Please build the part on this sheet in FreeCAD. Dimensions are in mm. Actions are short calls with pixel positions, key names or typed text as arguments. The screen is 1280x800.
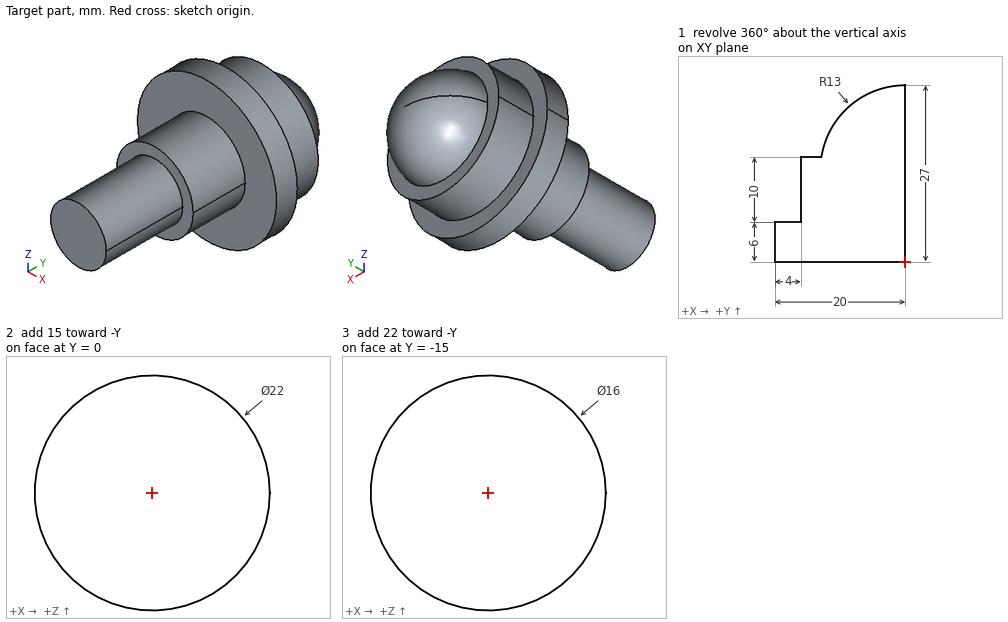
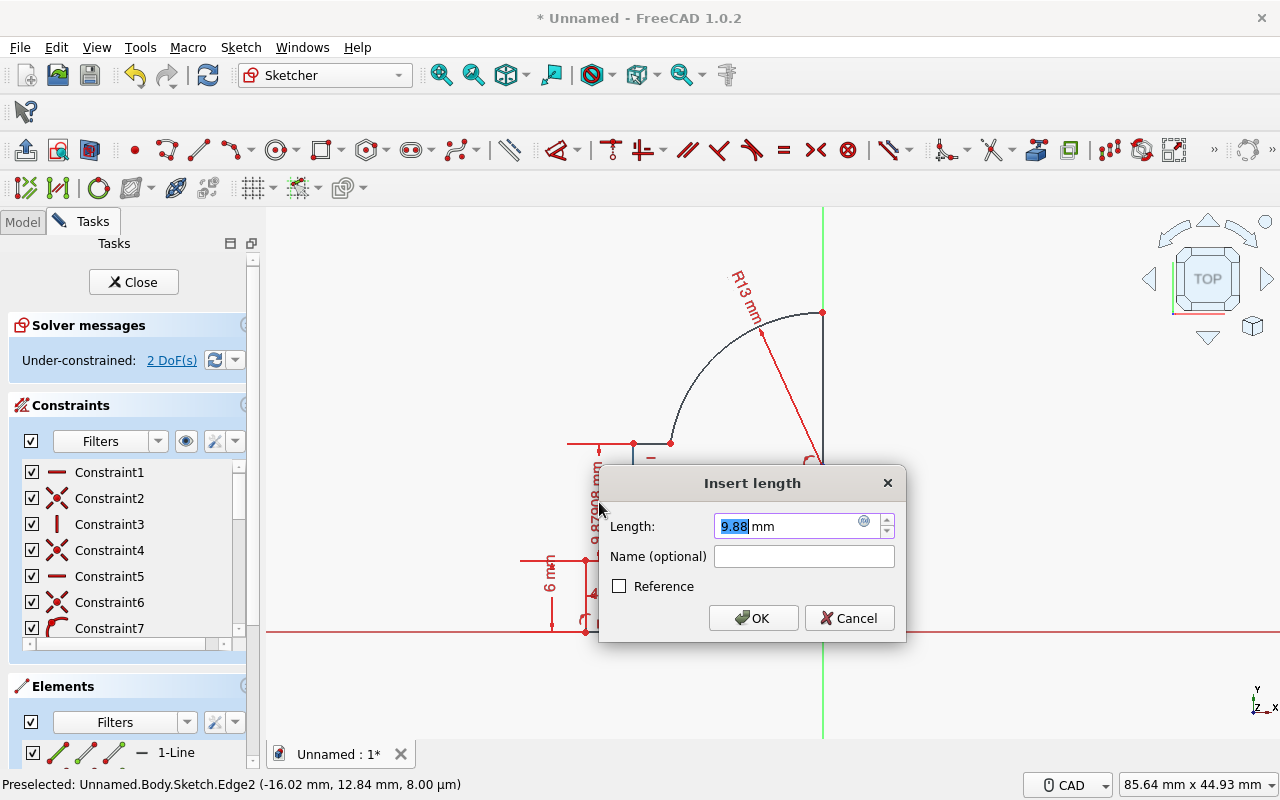
text(10)
key(Return)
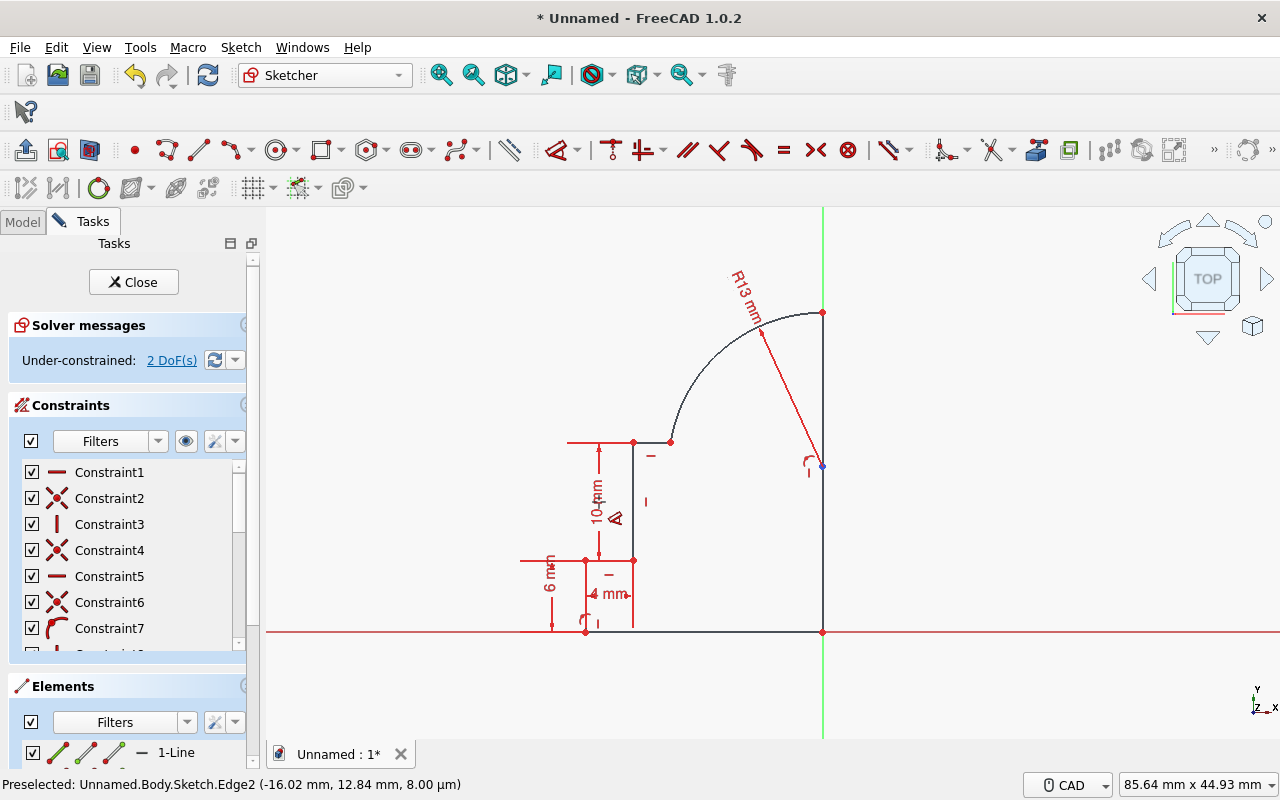
click(657, 632)
click(704, 666)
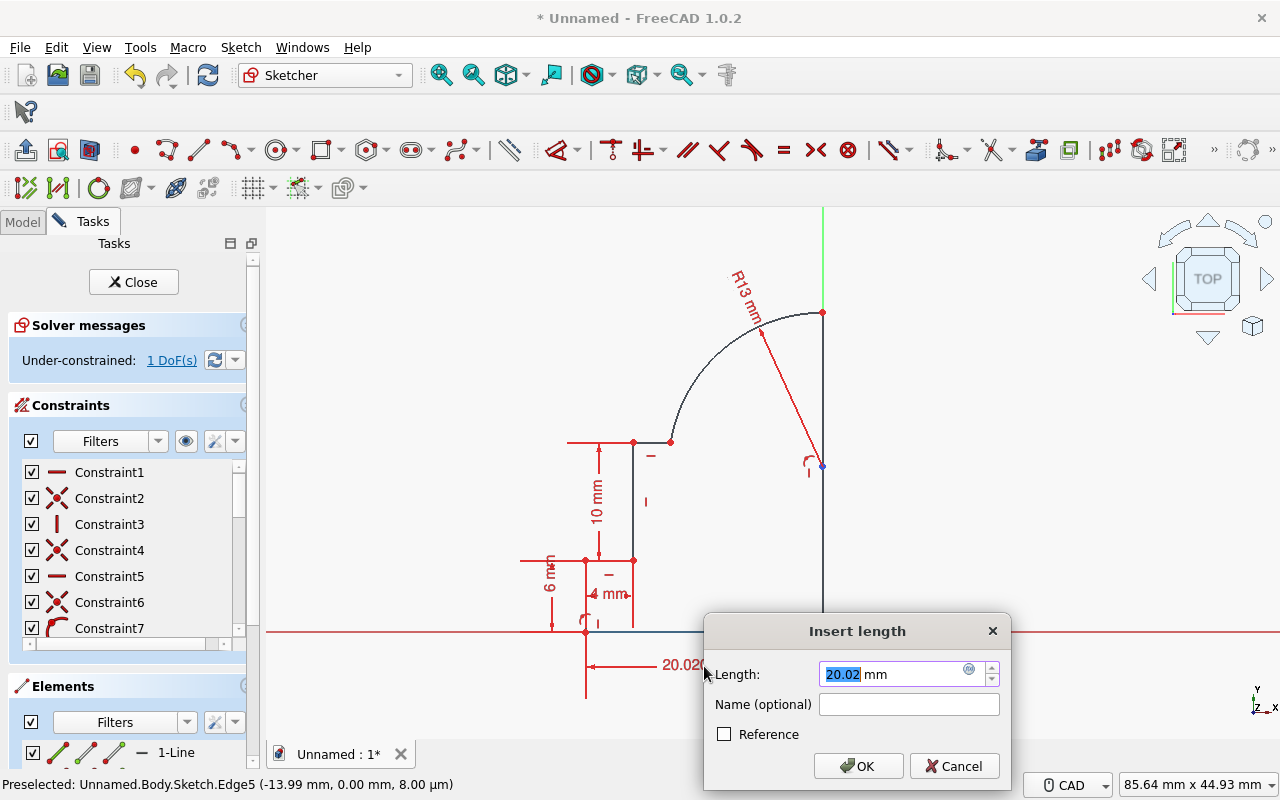
text(20)
key(Return)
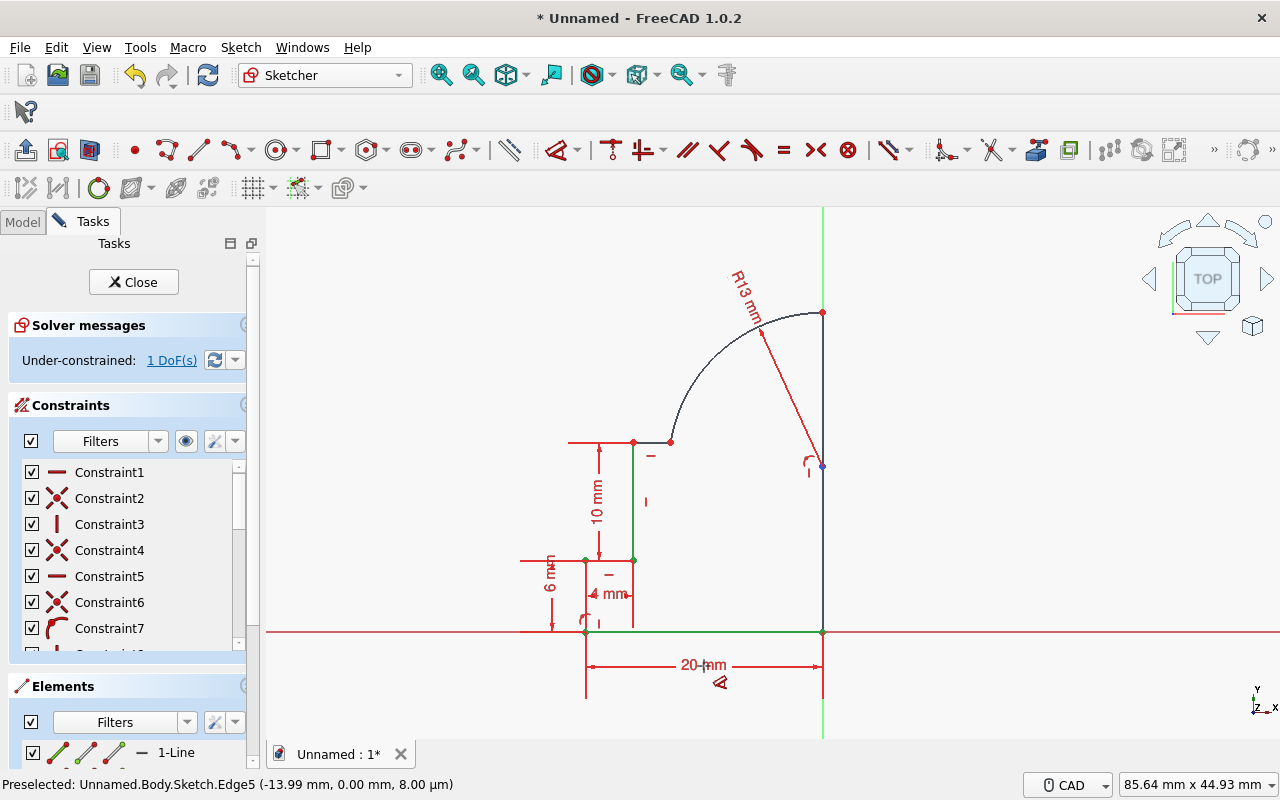
click(823, 536)
click(857, 472)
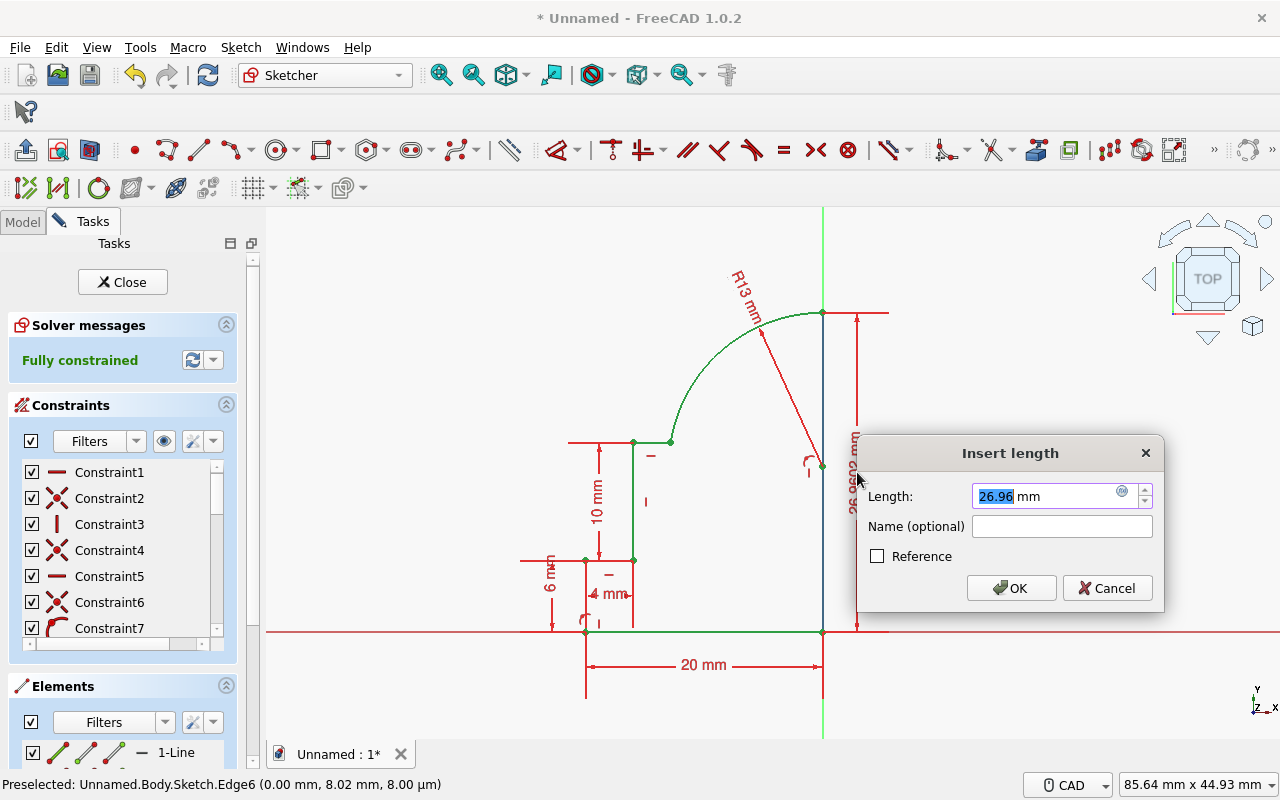
text(27)
key(Return)
key(Escape)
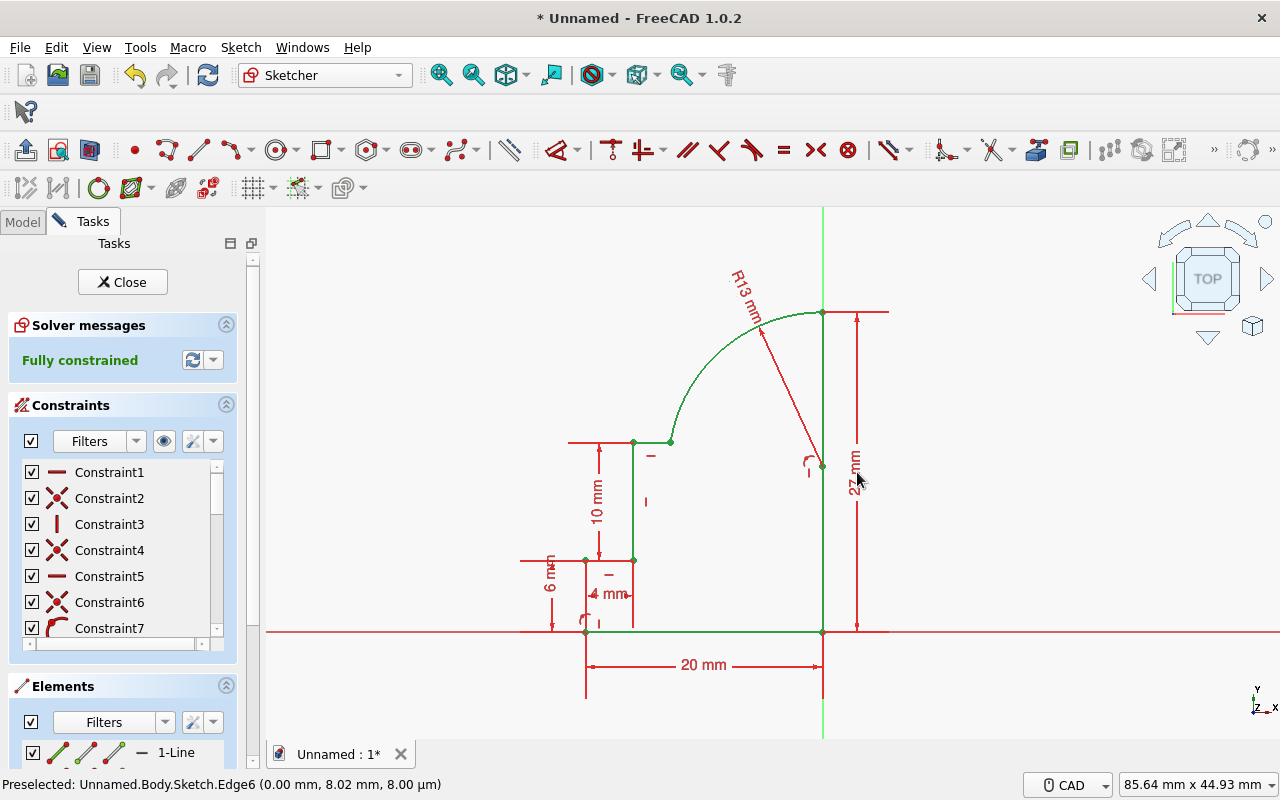
click(123, 282)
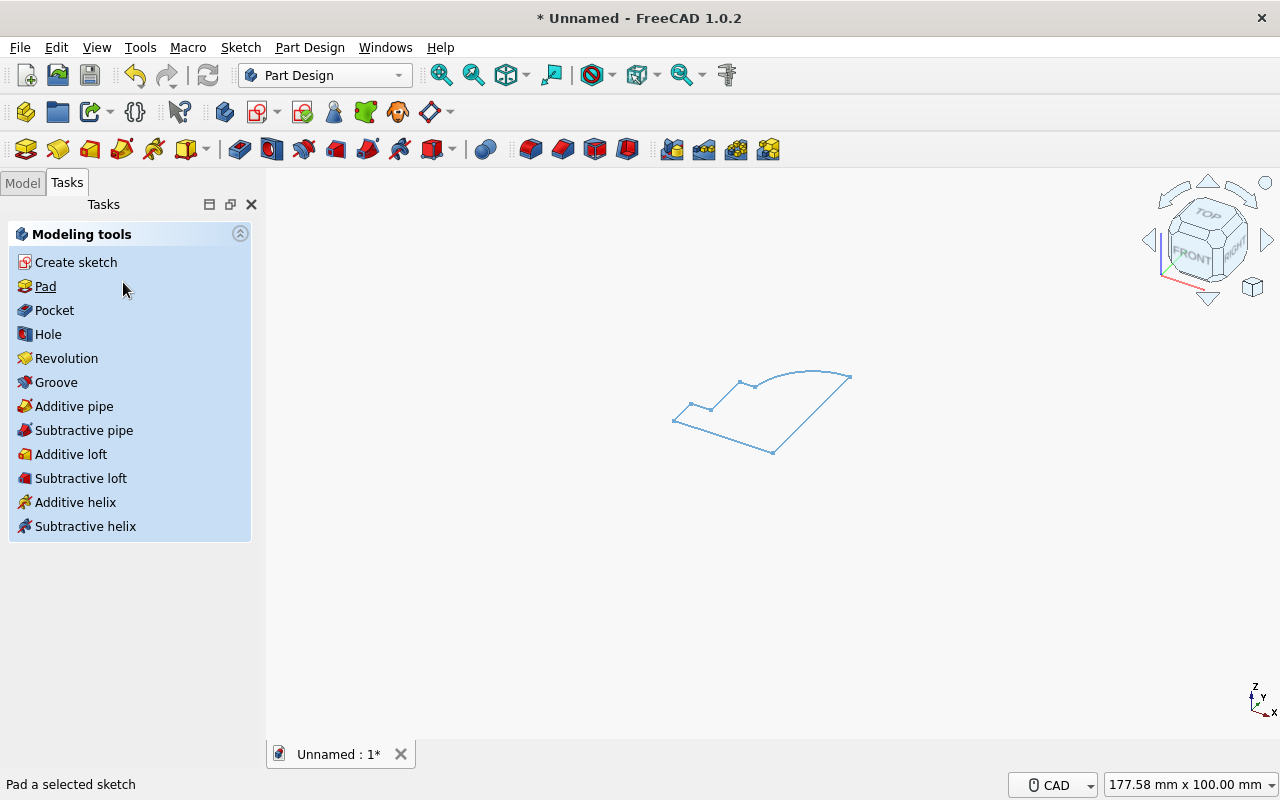
click(58, 150)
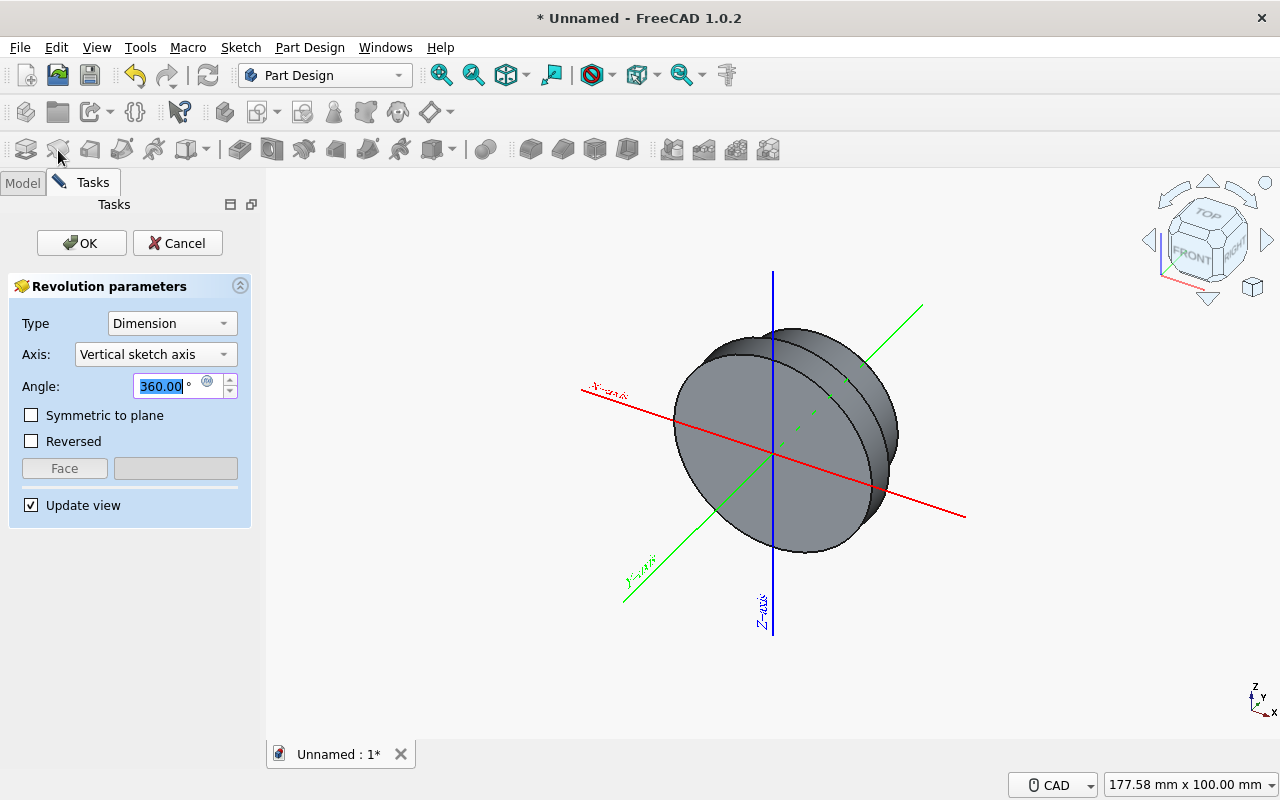
click(82, 243)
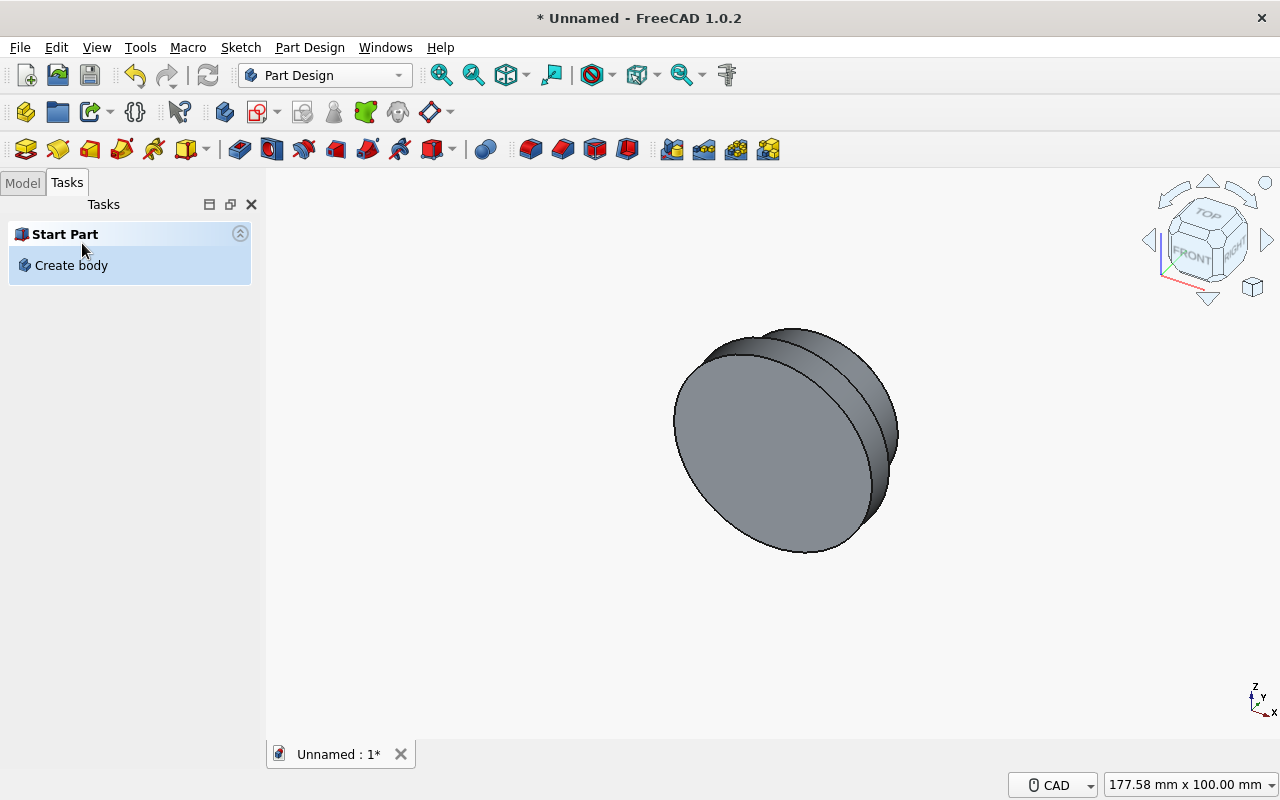
click(773, 452)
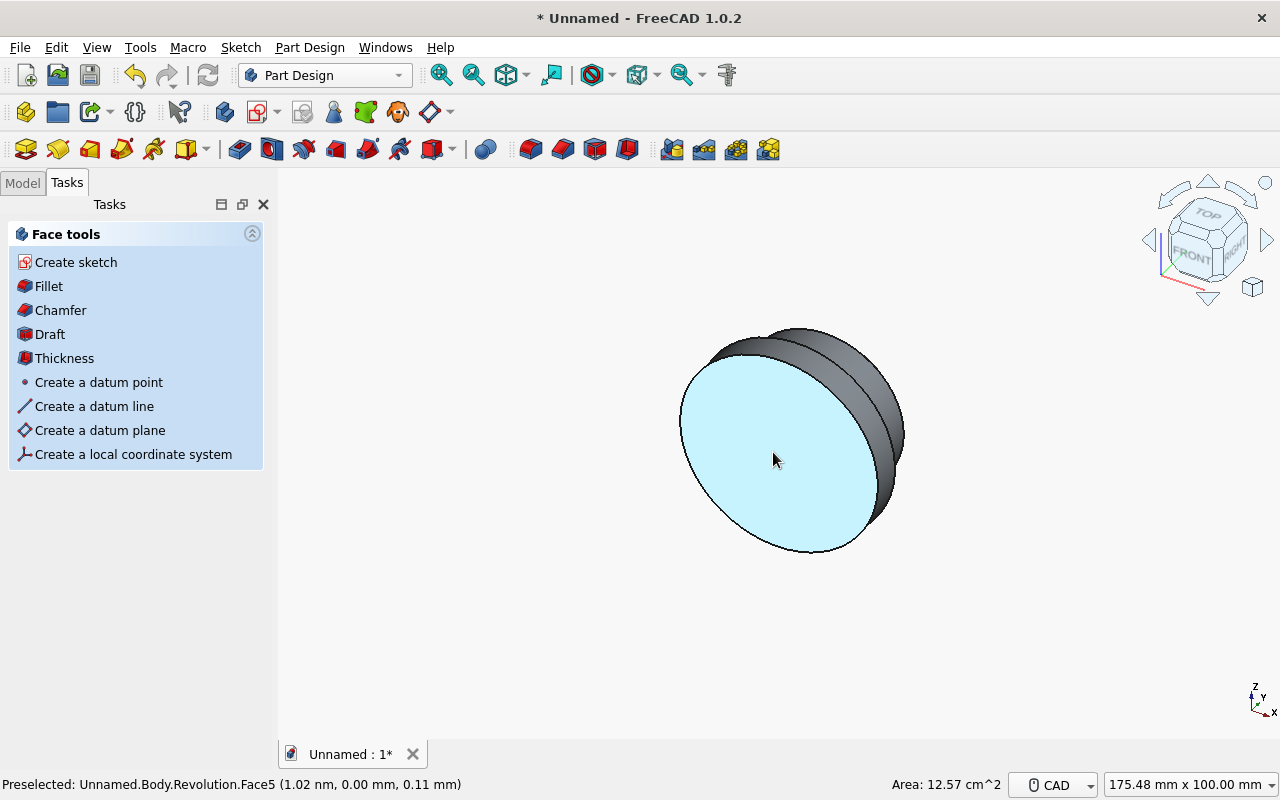
click(258, 112)